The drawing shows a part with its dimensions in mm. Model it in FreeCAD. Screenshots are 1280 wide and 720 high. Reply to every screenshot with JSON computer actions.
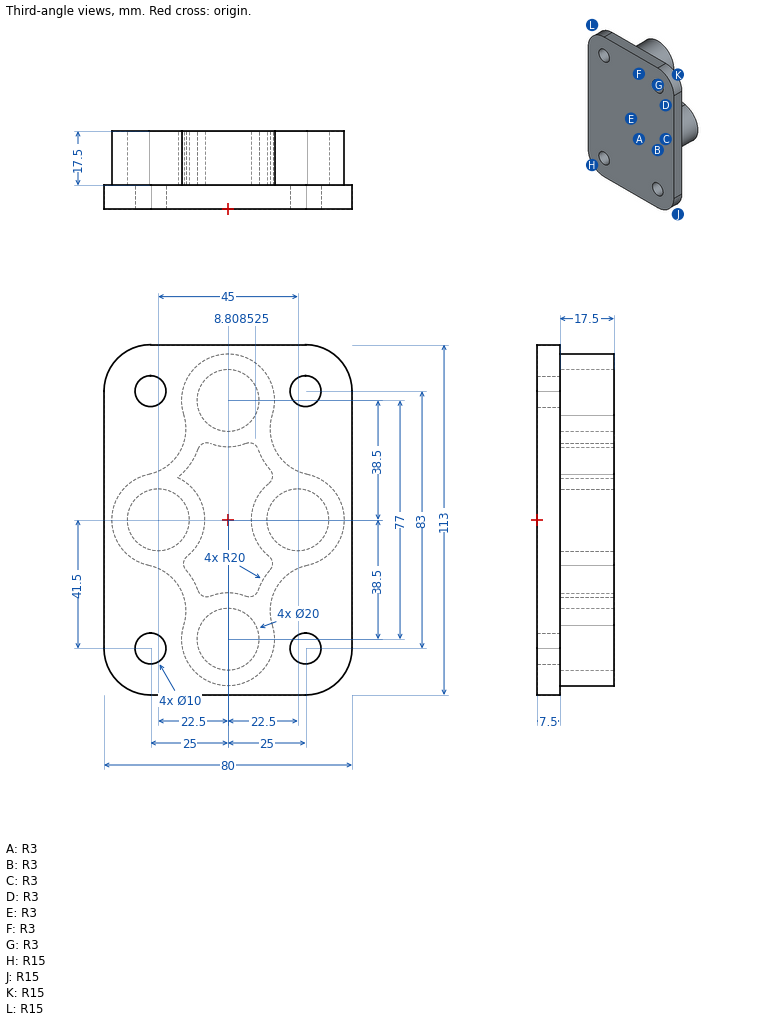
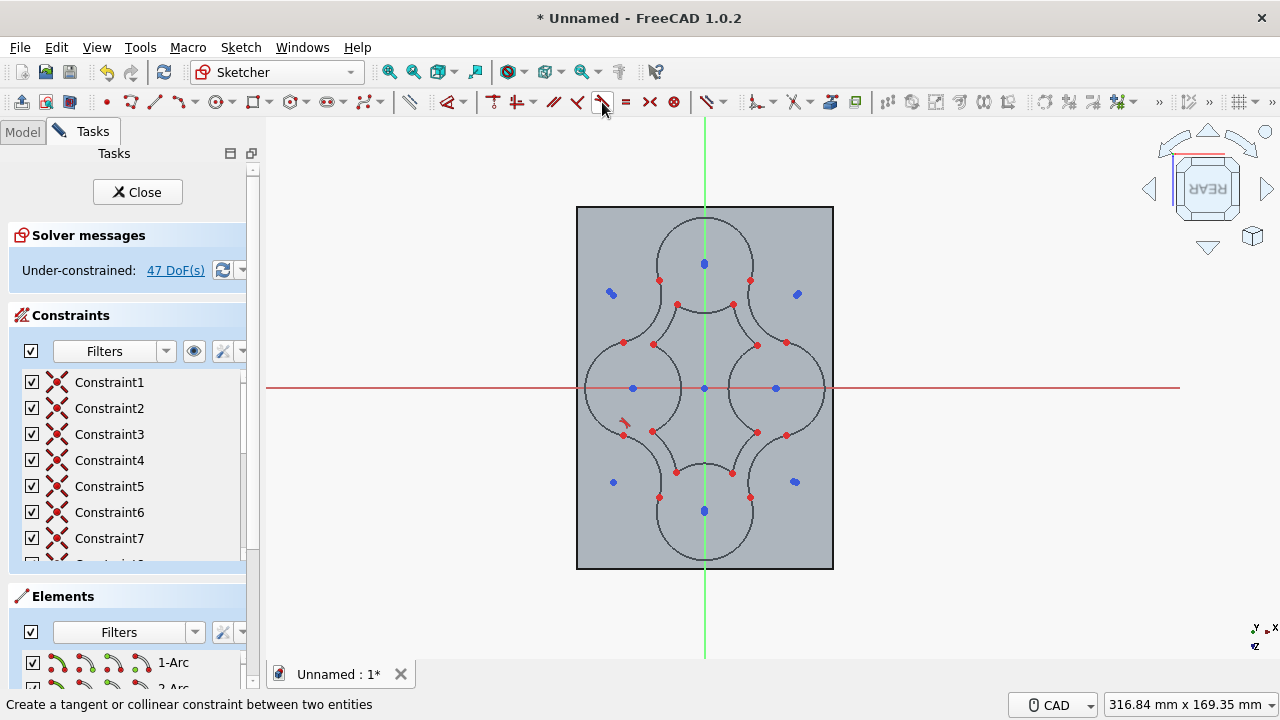
{"action": "left_click", "coordinate": [592, 364]}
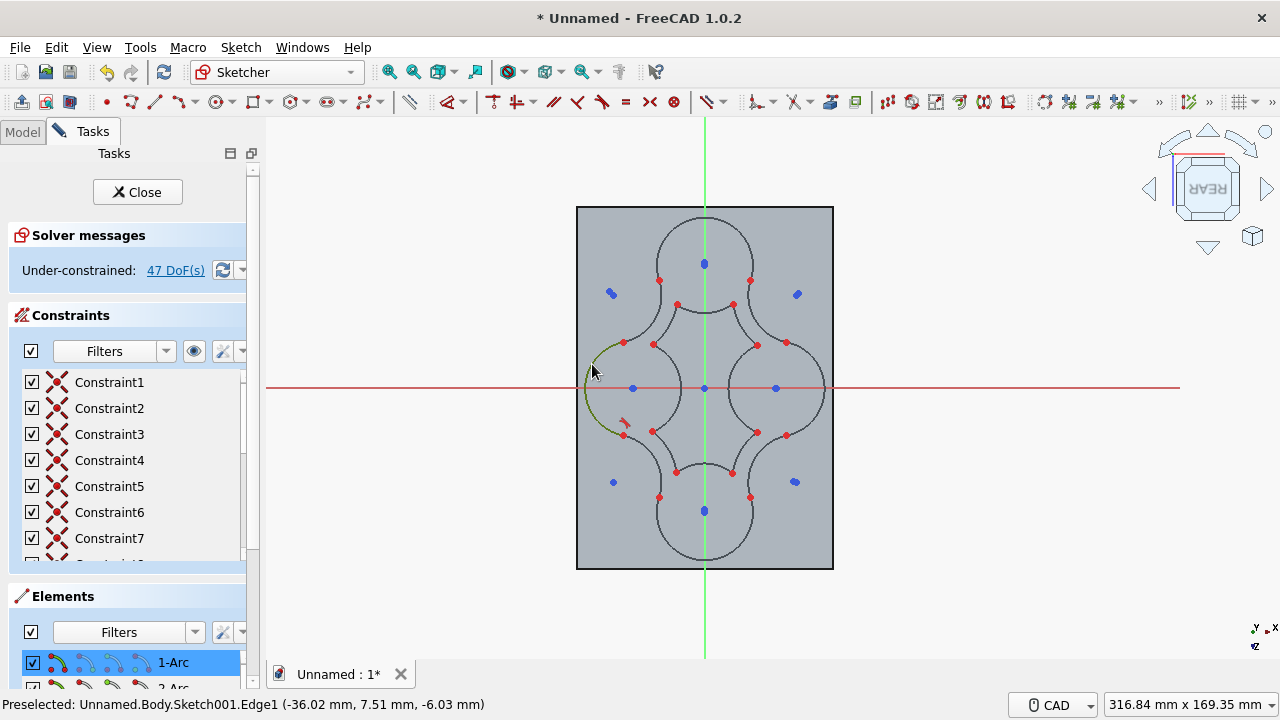
{"action": "left_click", "coordinate": [645, 332]}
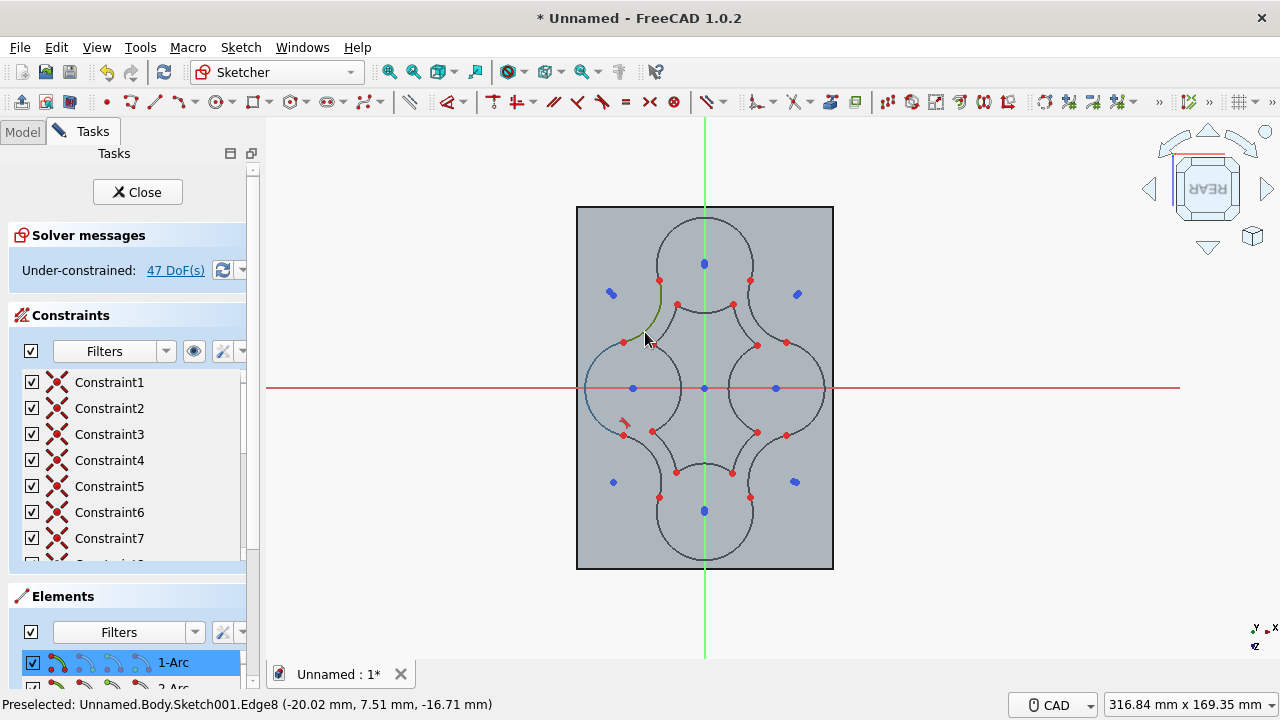
{"action": "key", "text": "t"}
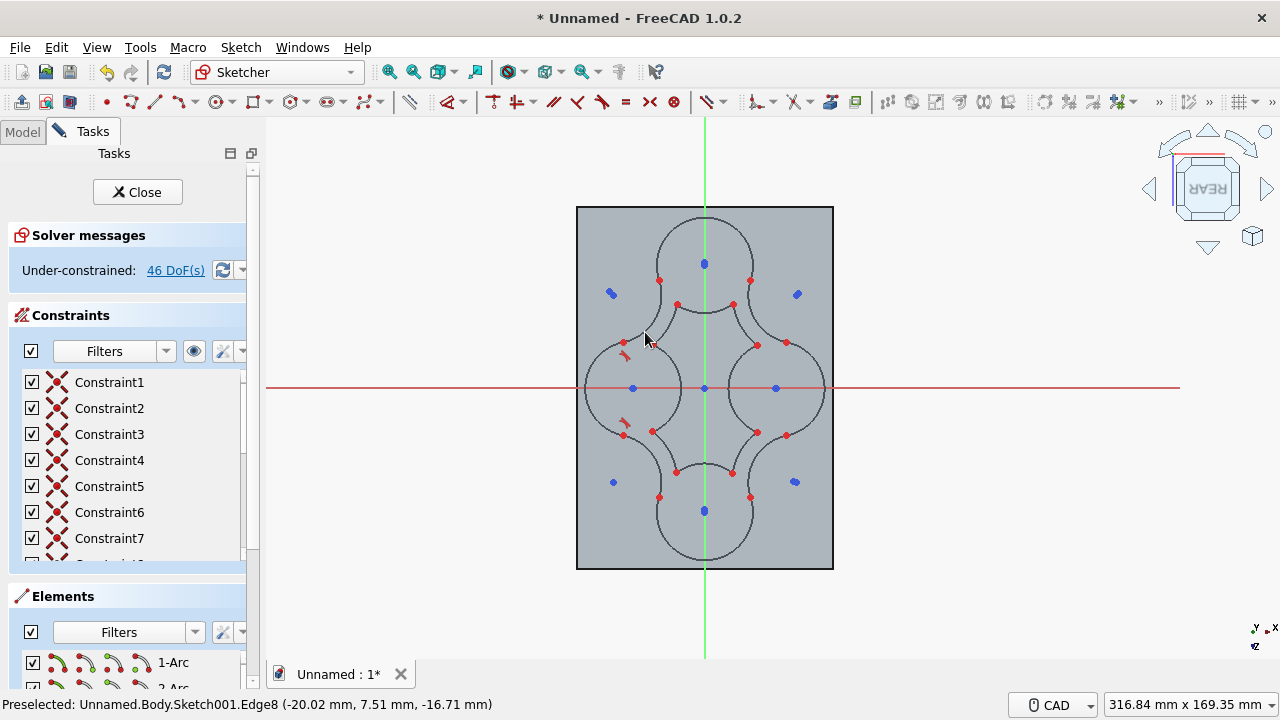
{"action": "left_click", "coordinate": [661, 474]}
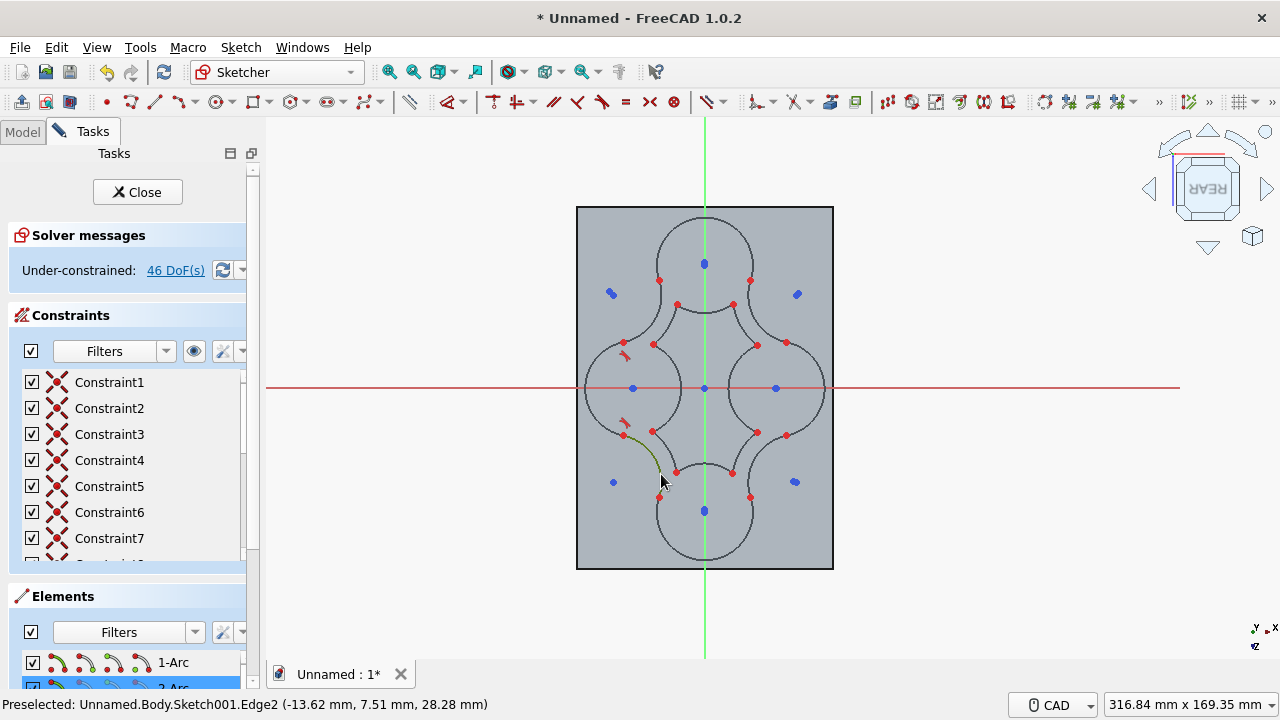
{"action": "left_click", "coordinate": [672, 547]}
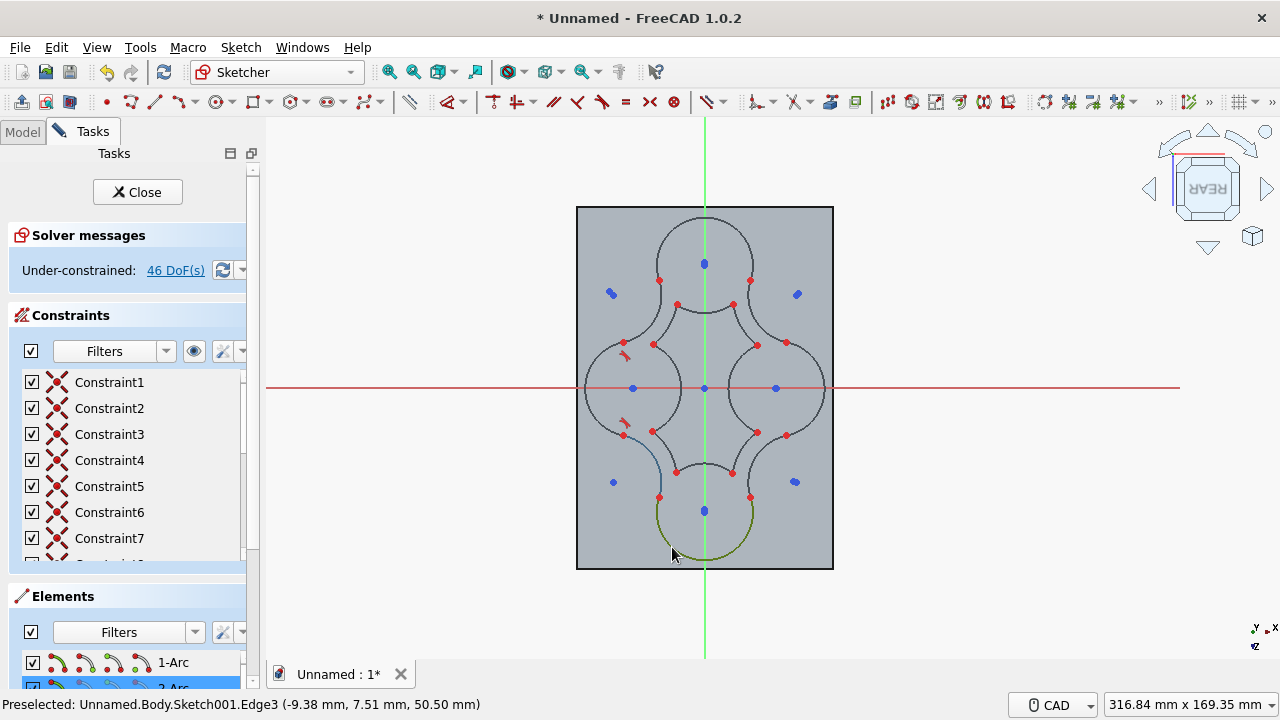
{"action": "left_click", "coordinate": [602, 102]}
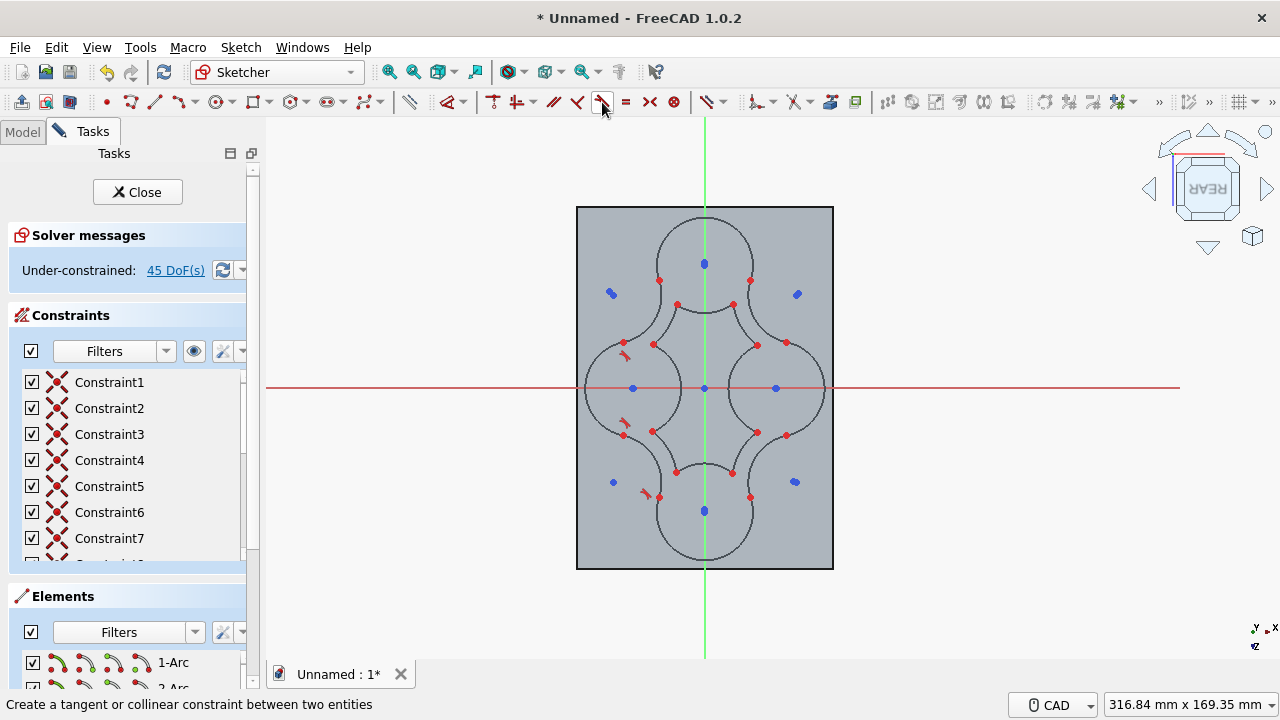
{"action": "left_click", "coordinate": [672, 547]}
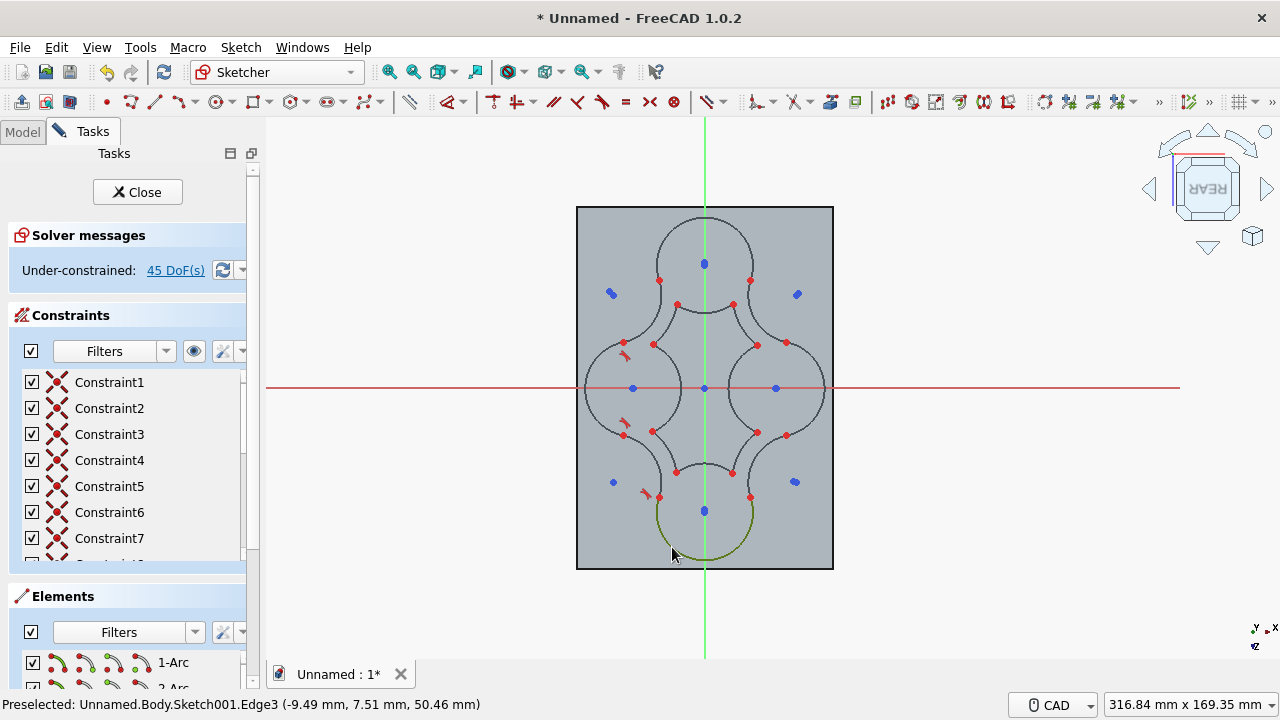
{"action": "left_click", "coordinate": [765, 446]}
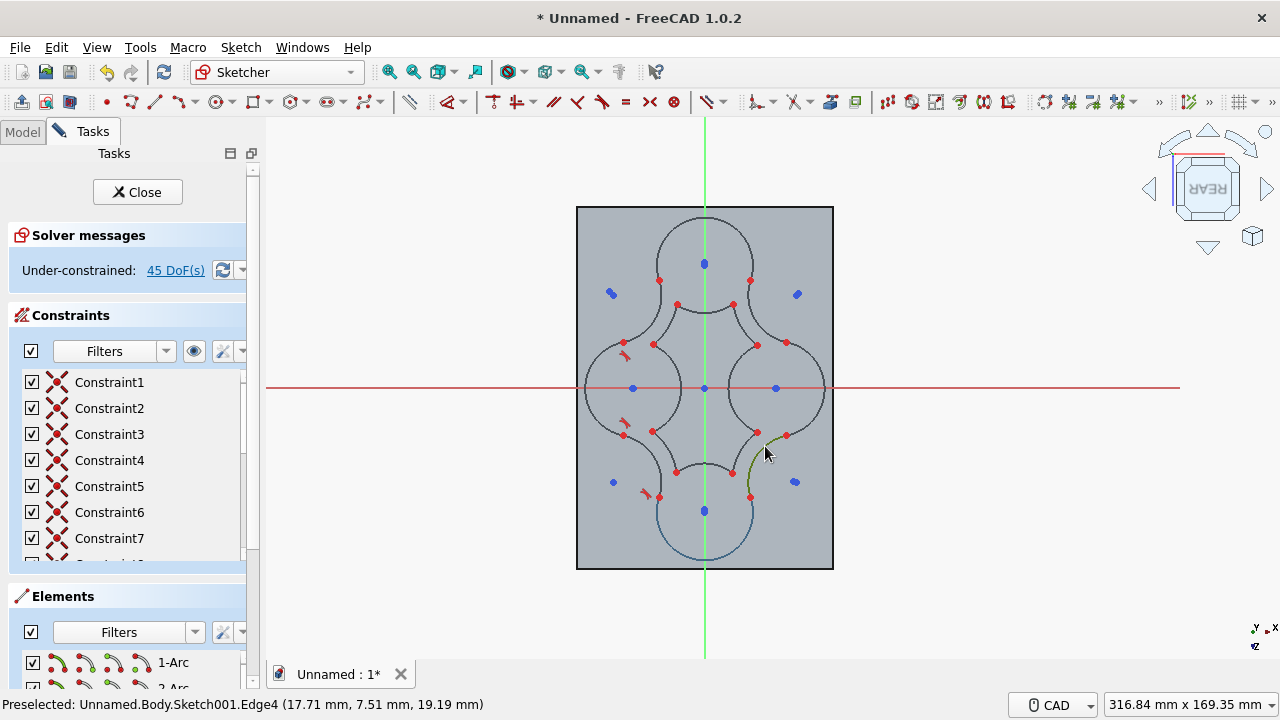
{"action": "left_click", "coordinate": [602, 102]}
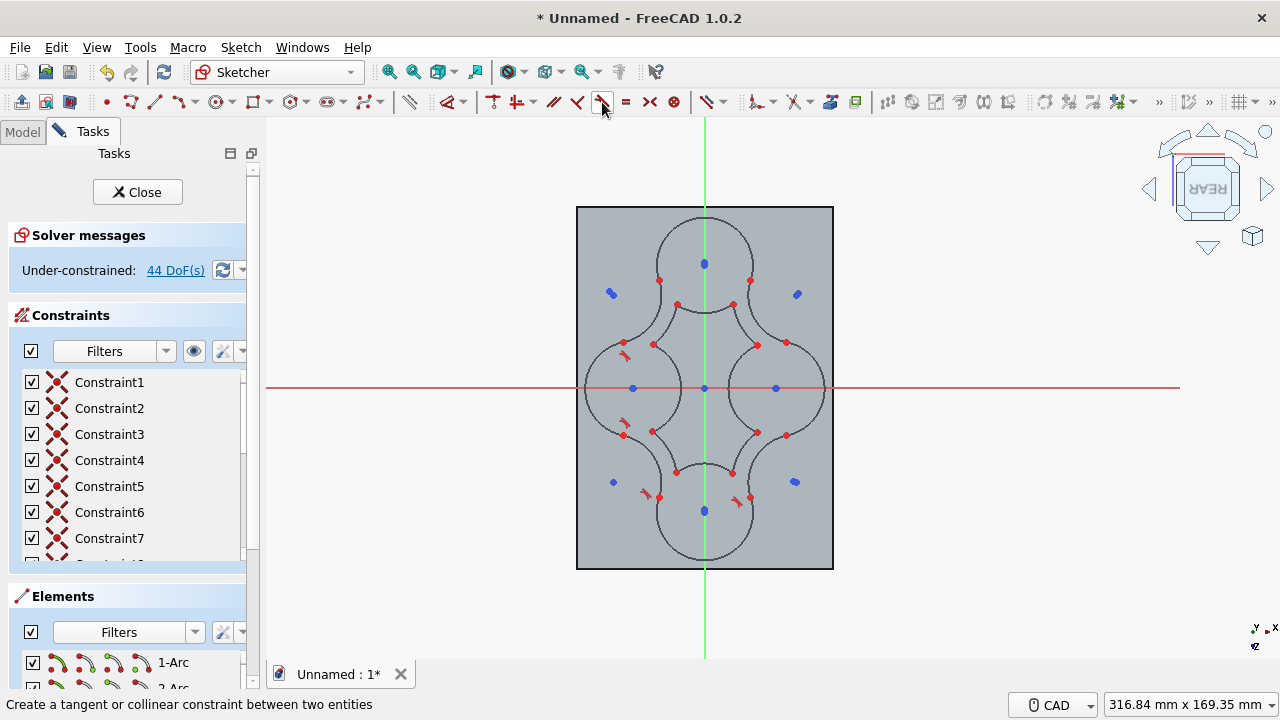
{"action": "left_click", "coordinate": [765, 446]}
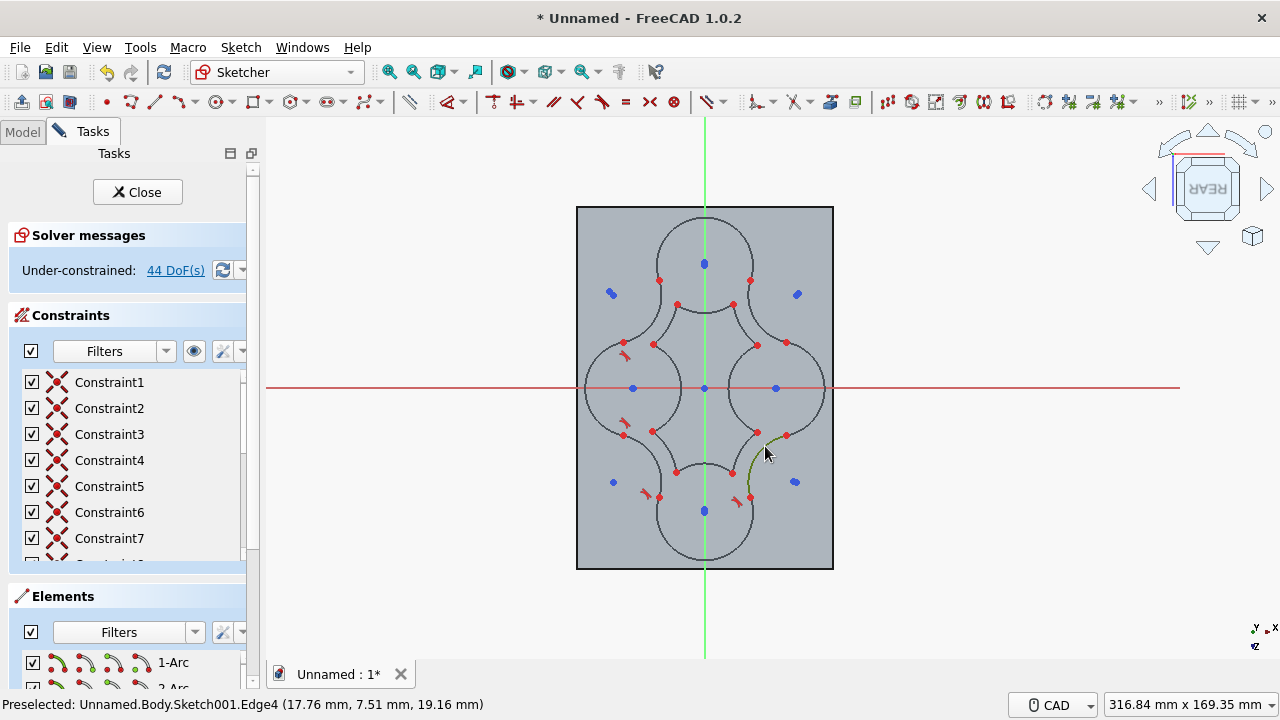
{"action": "left_click", "coordinate": [818, 414]}